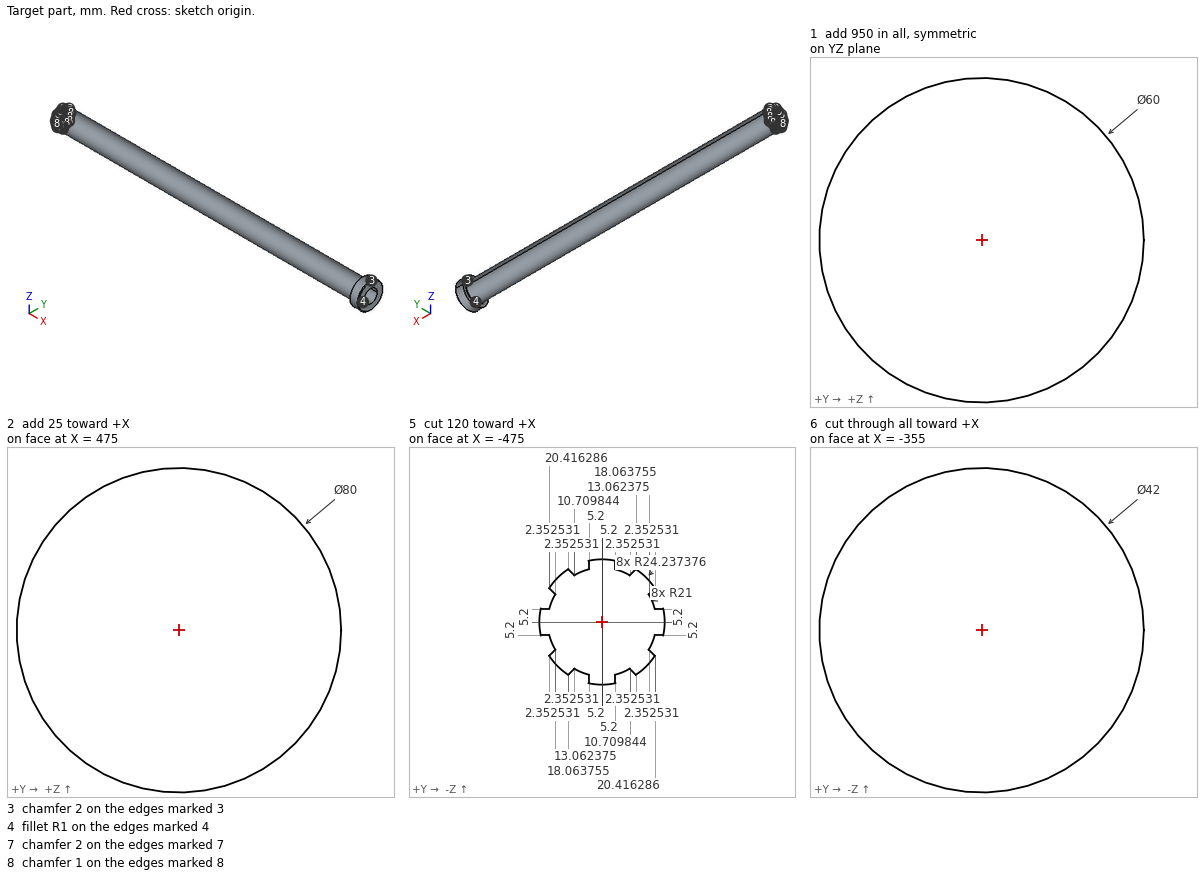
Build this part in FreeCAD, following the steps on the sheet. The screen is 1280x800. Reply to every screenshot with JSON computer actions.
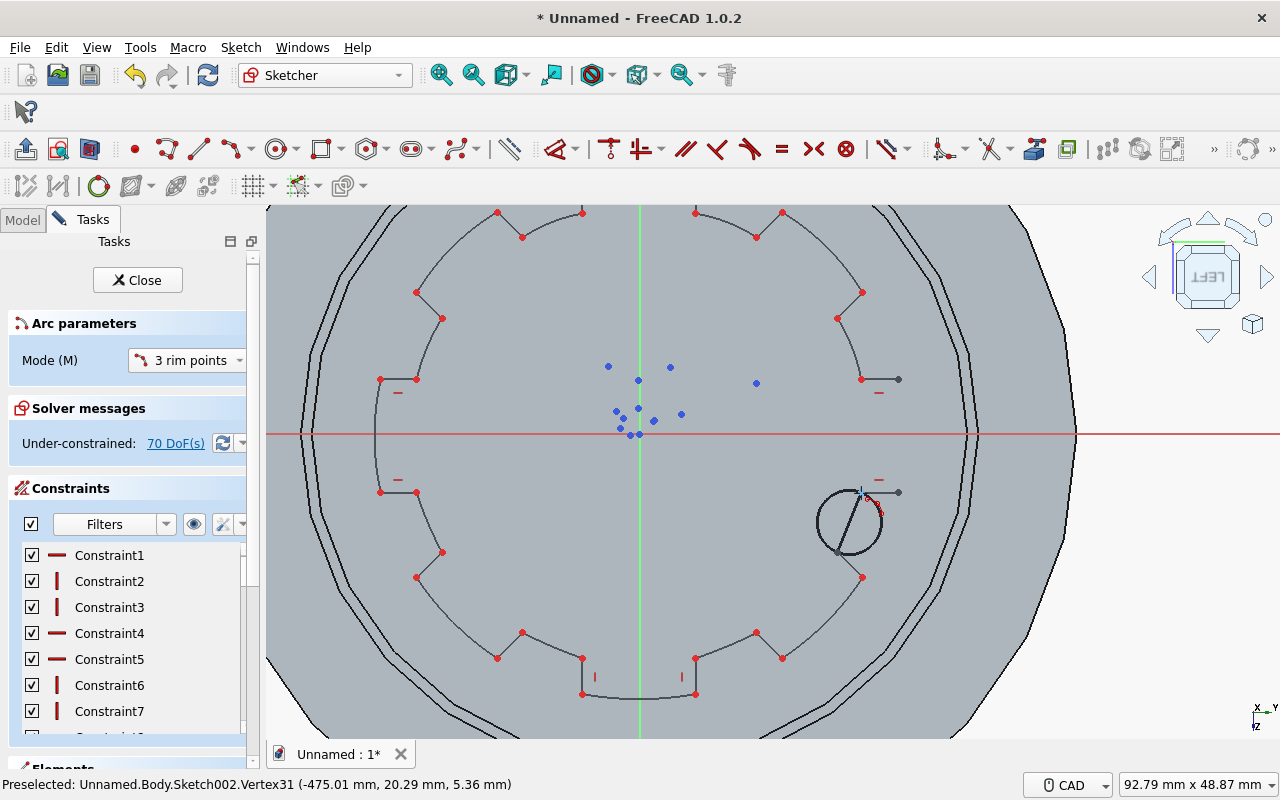
{"action": "scroll", "coordinate": [852, 522], "scroll_direction": "up", "scroll_amount": 10}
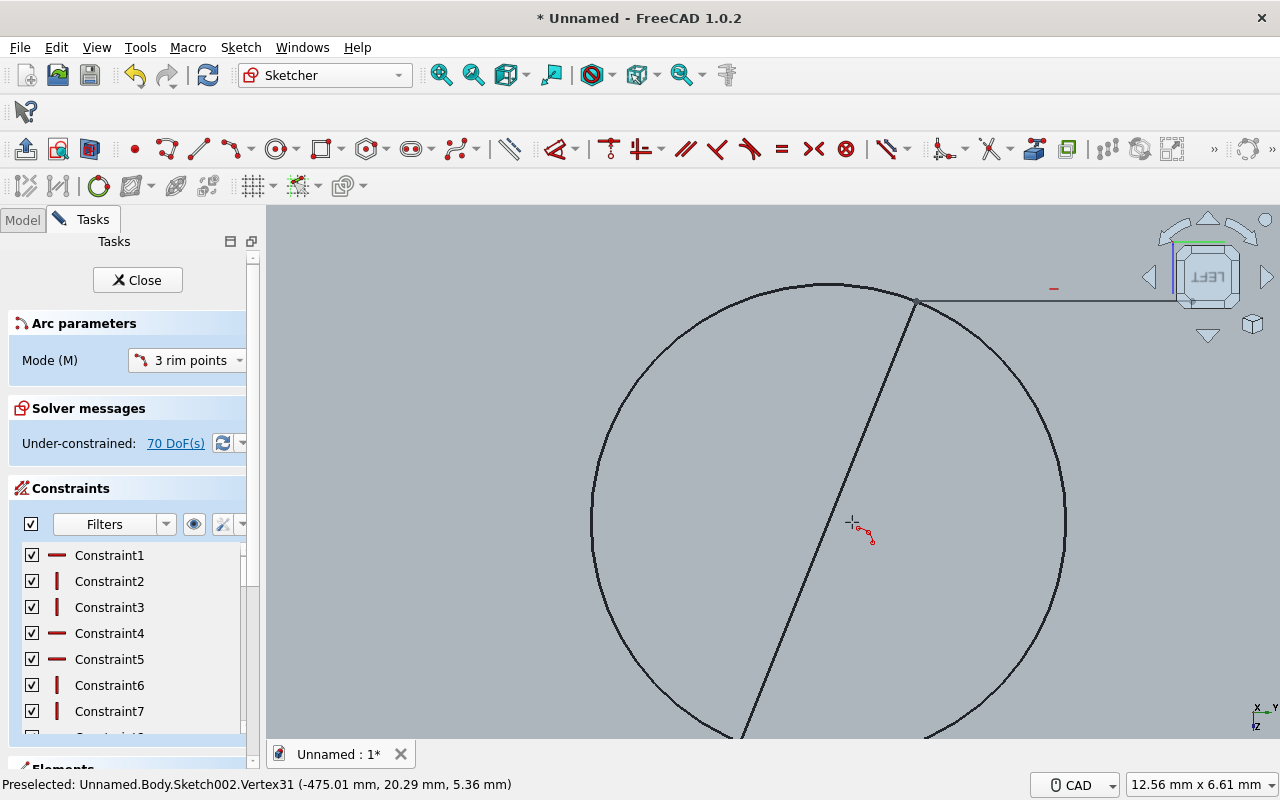
{"action": "left_click", "coordinate": [845, 518]}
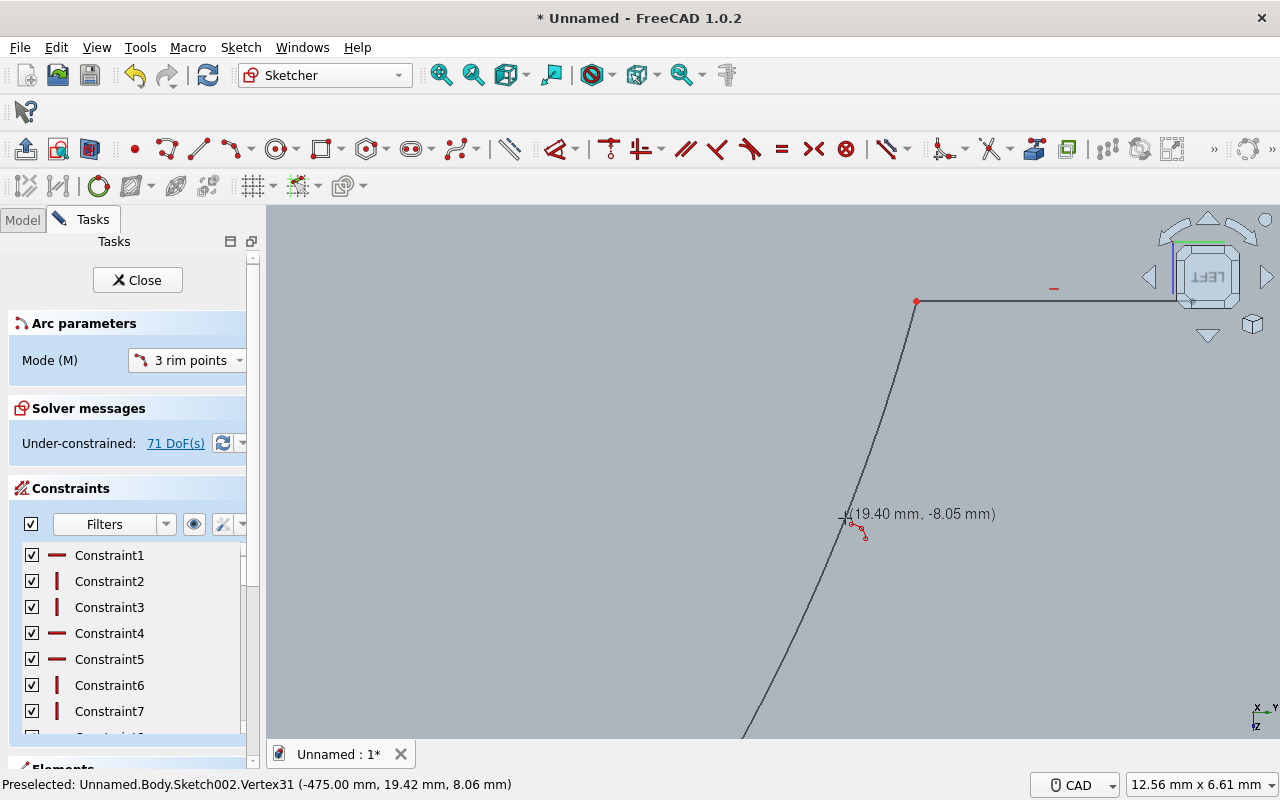
{"action": "scroll", "coordinate": [847, 532], "scroll_direction": "down", "scroll_amount": 12}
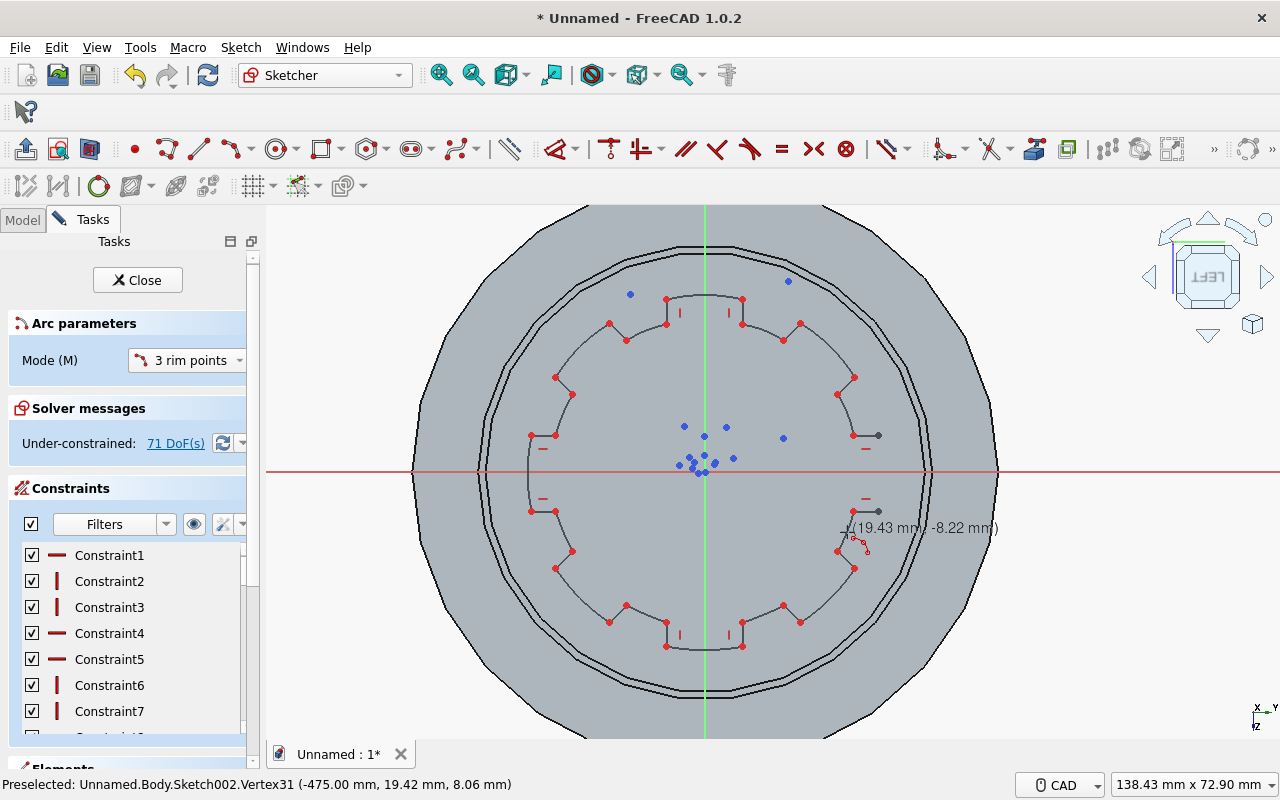
{"action": "scroll", "coordinate": [879, 510], "scroll_direction": "up", "scroll_amount": 2}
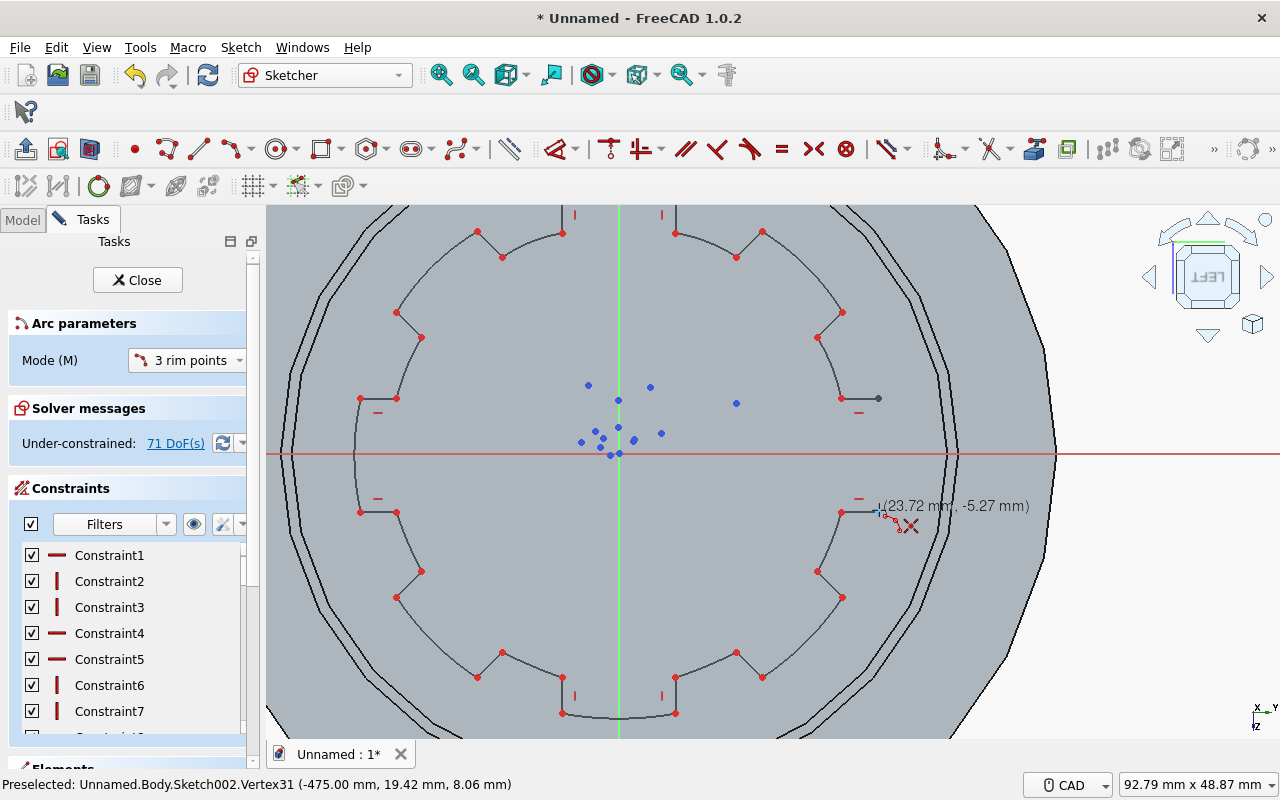
{"action": "left_click", "coordinate": [878, 512]}
{"action": "left_click", "coordinate": [878, 399]}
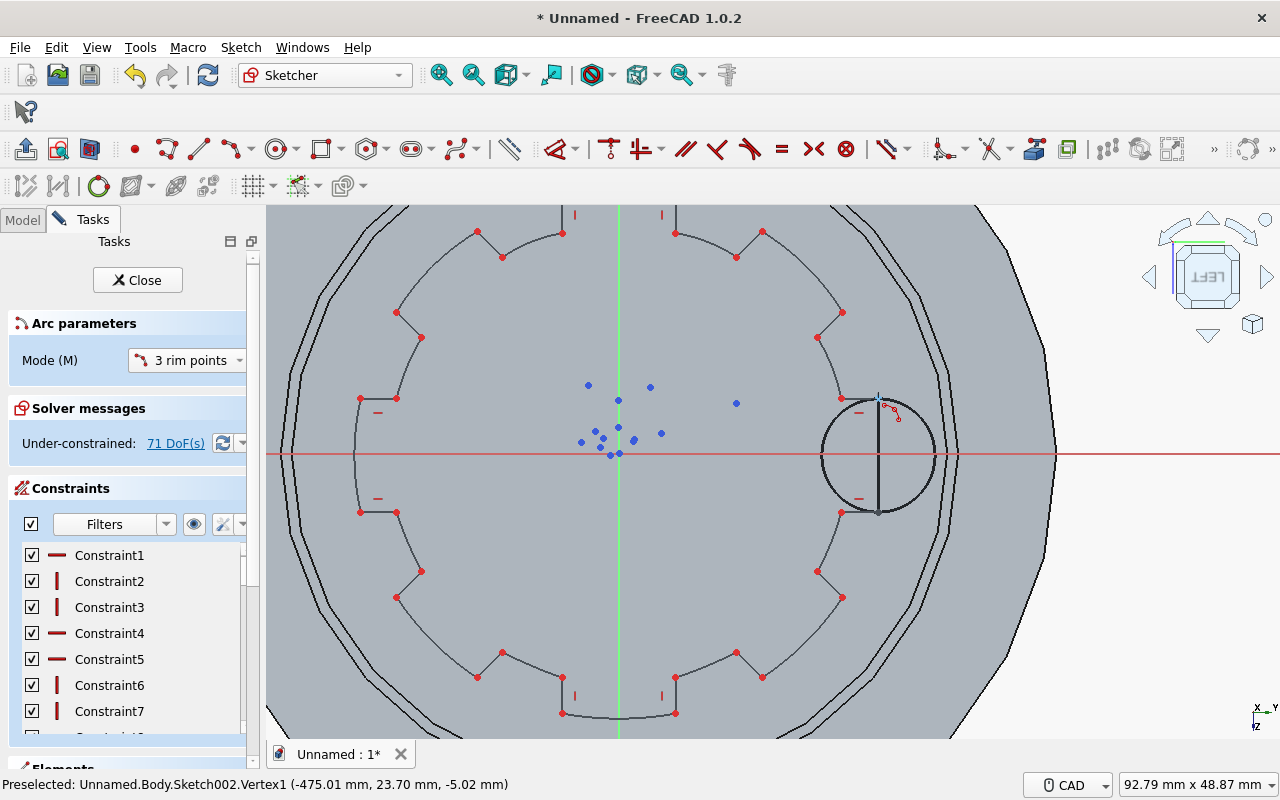
{"action": "scroll", "coordinate": [884, 465], "scroll_direction": "up", "scroll_amount": 5}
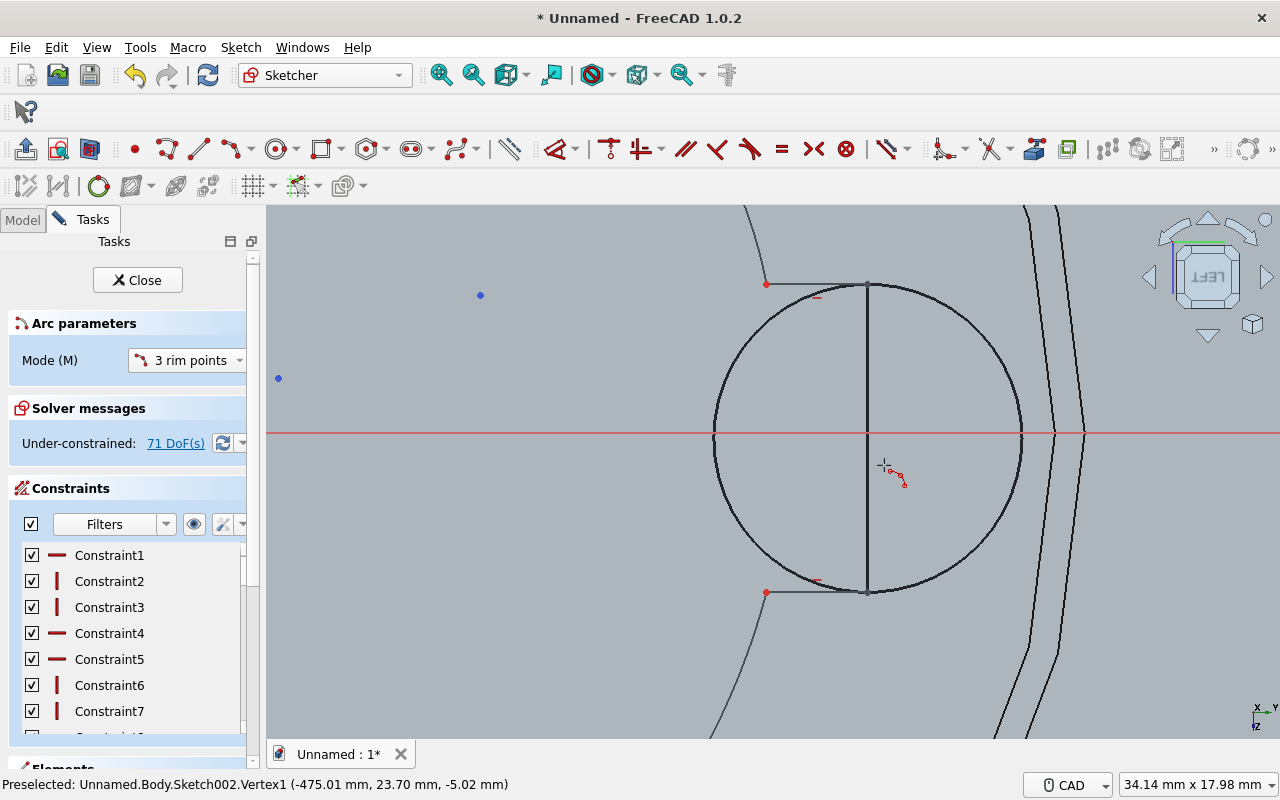
{"action": "left_click", "coordinate": [883, 464]}
{"action": "key", "text": "Escape"}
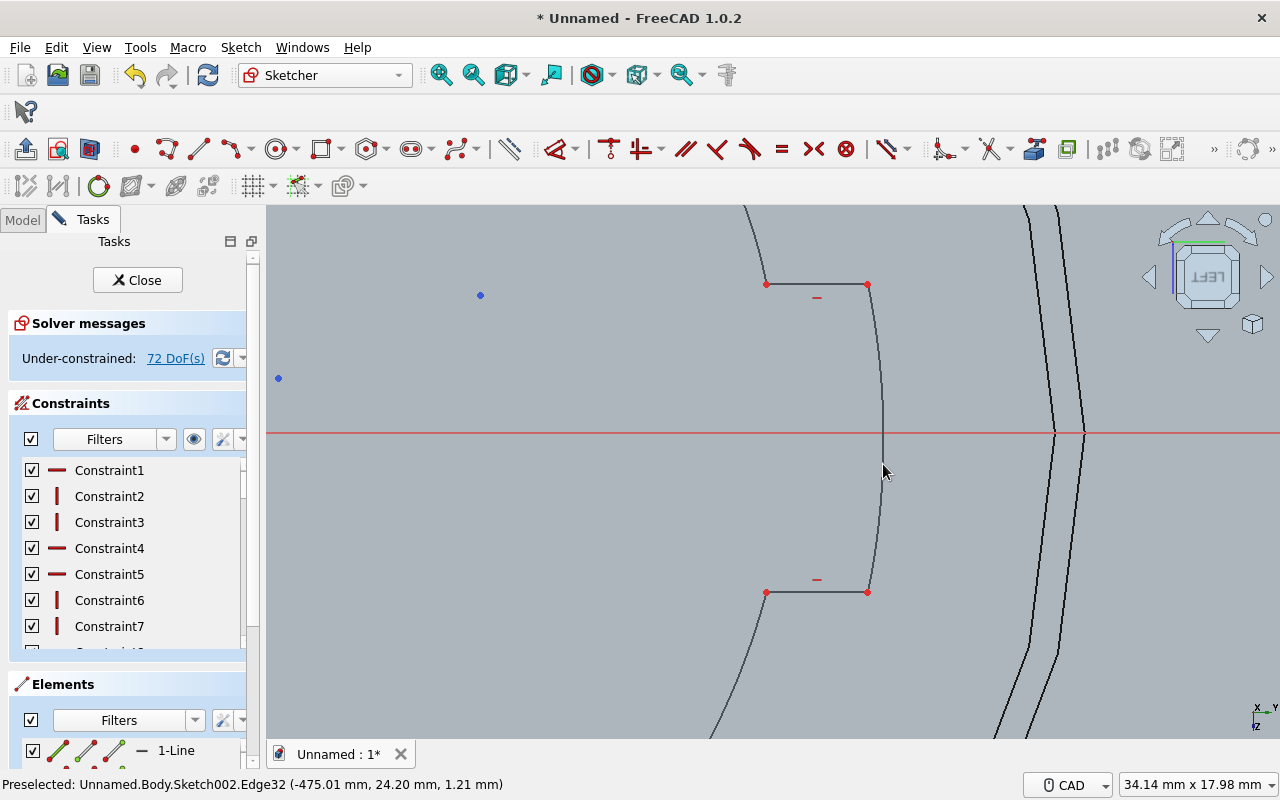
{"action": "left_click", "coordinate": [758, 249]}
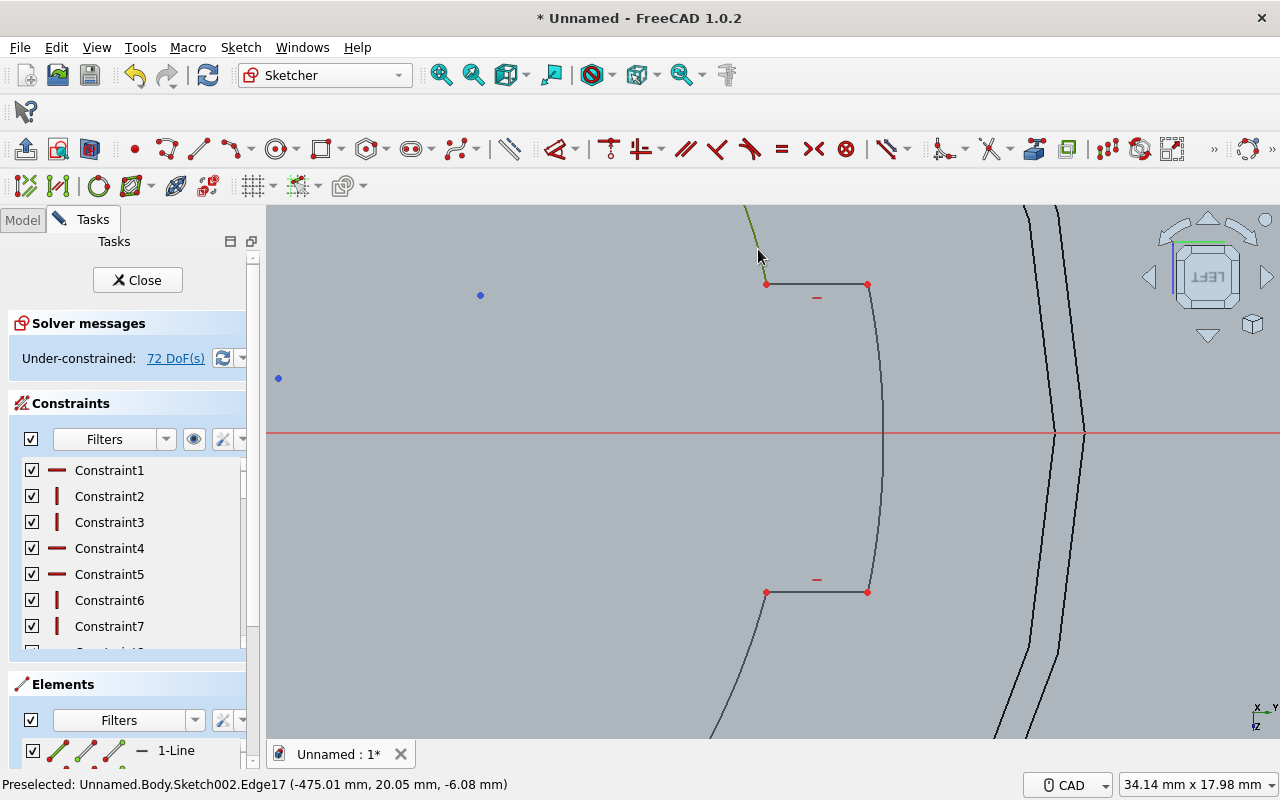
{"action": "scroll", "coordinate": [881, 485], "scroll_direction": "down", "scroll_amount": 7}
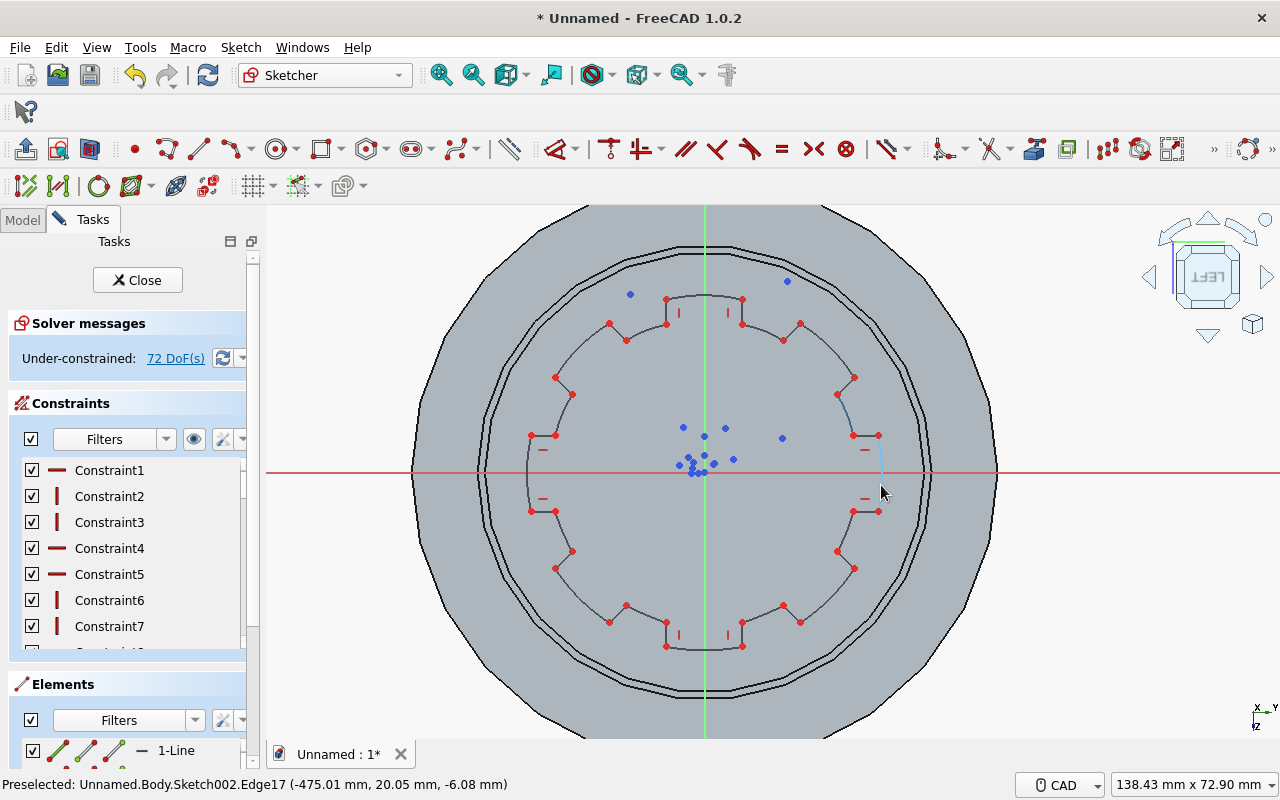
{"action": "left_click", "coordinate": [841, 359]}